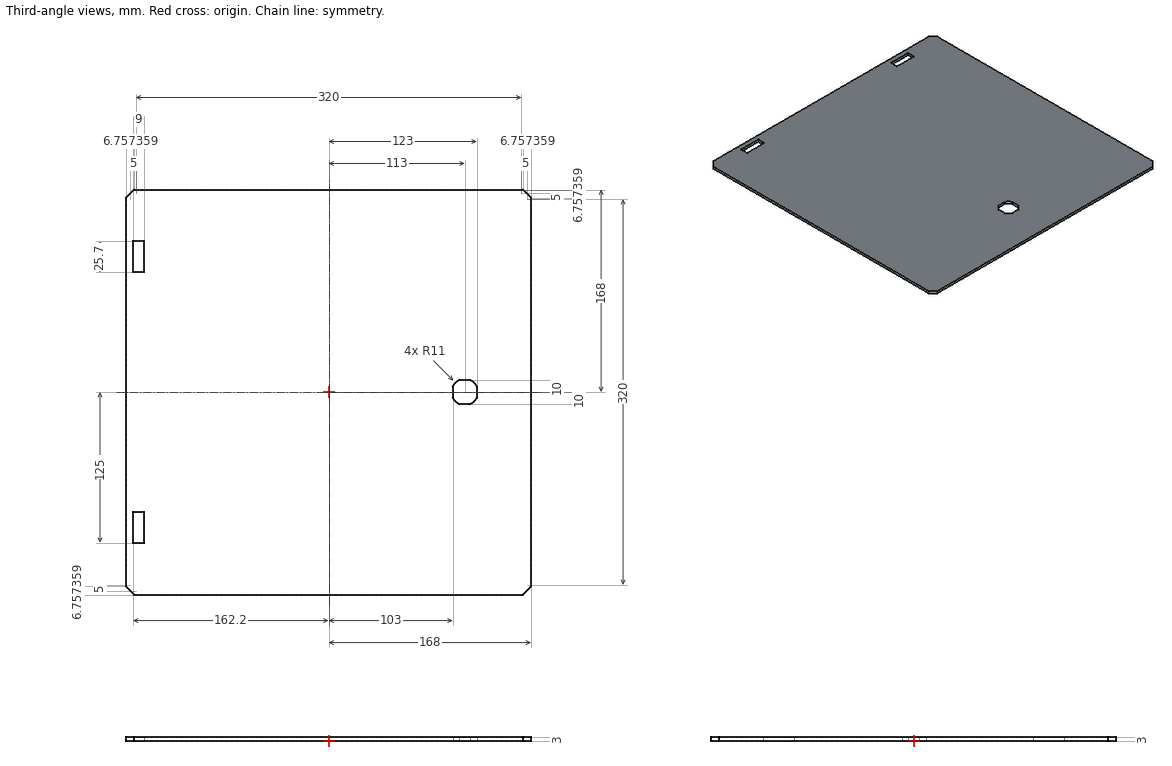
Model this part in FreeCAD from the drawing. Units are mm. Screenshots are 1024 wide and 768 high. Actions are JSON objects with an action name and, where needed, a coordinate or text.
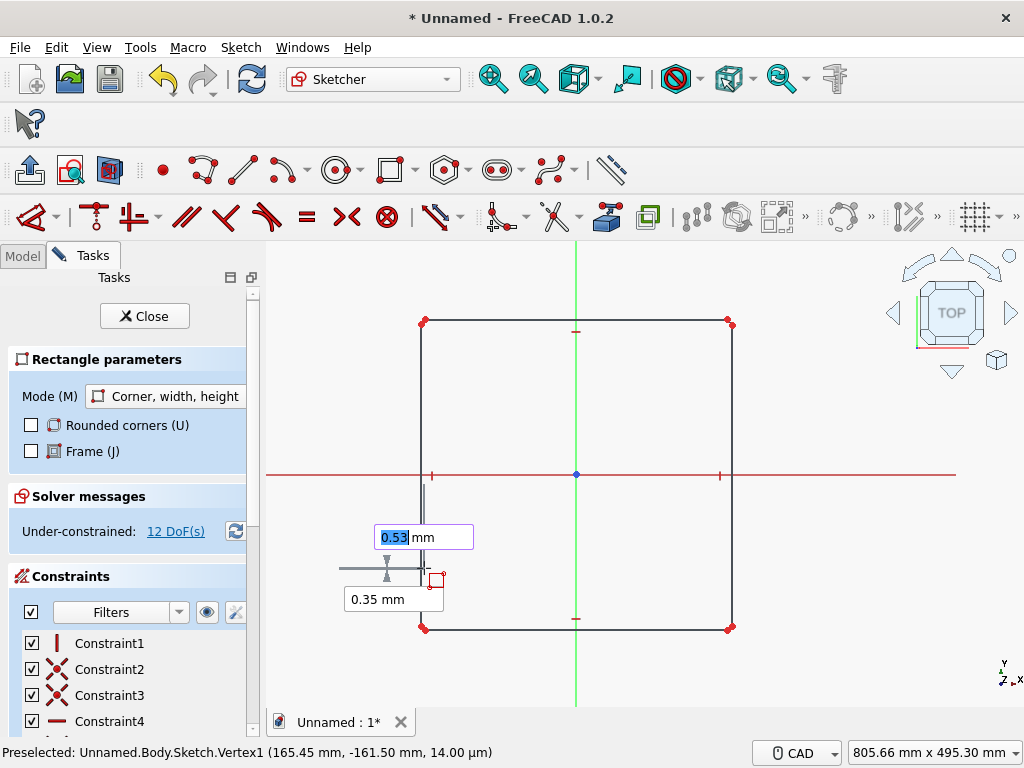
{"action": "scroll", "coordinate": [432, 592], "scroll_direction": "up", "scroll_amount": 2}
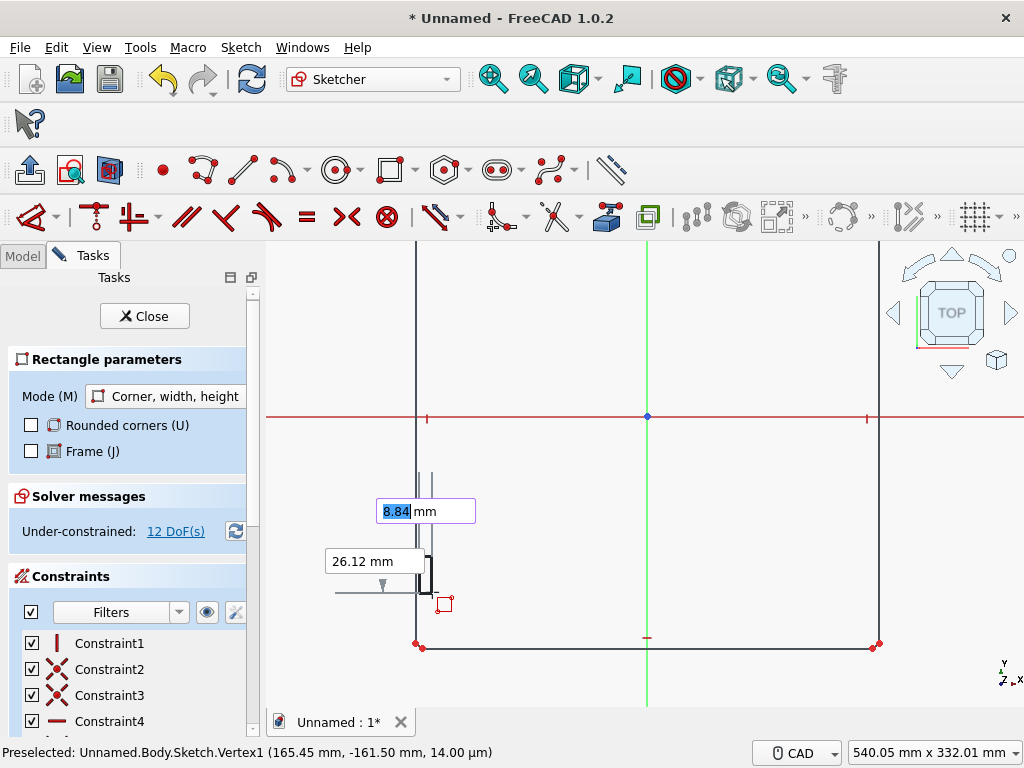
{"action": "left_click", "coordinate": [432, 592]}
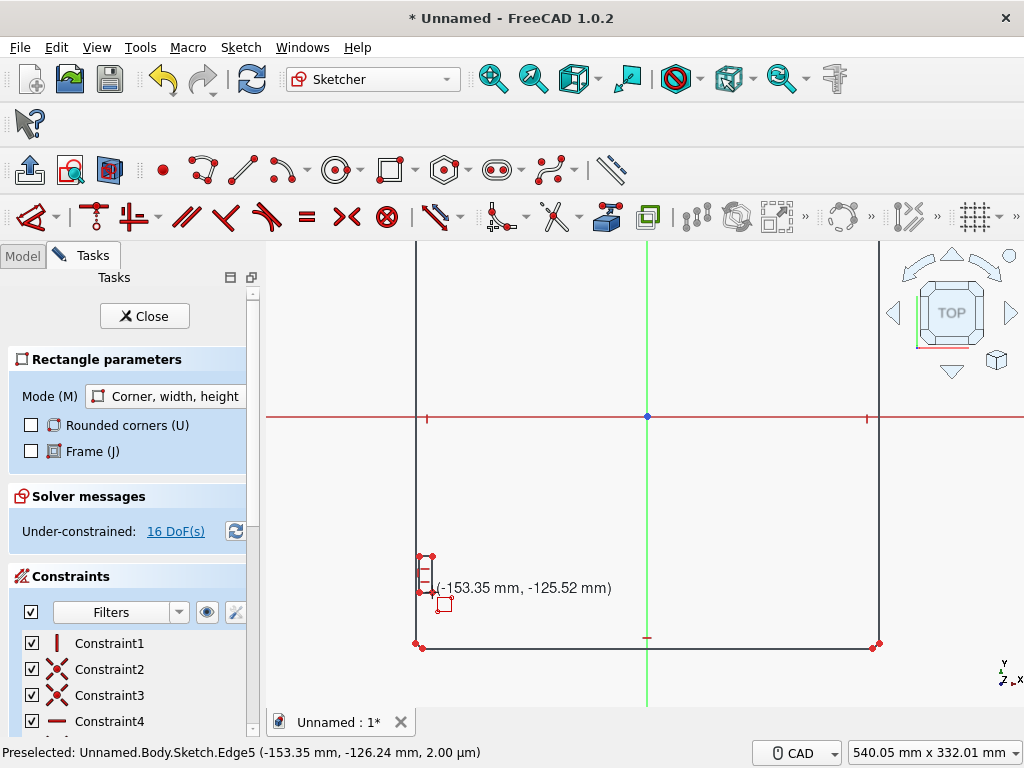
{"action": "scroll", "coordinate": [433, 590], "scroll_direction": "down", "scroll_amount": 2}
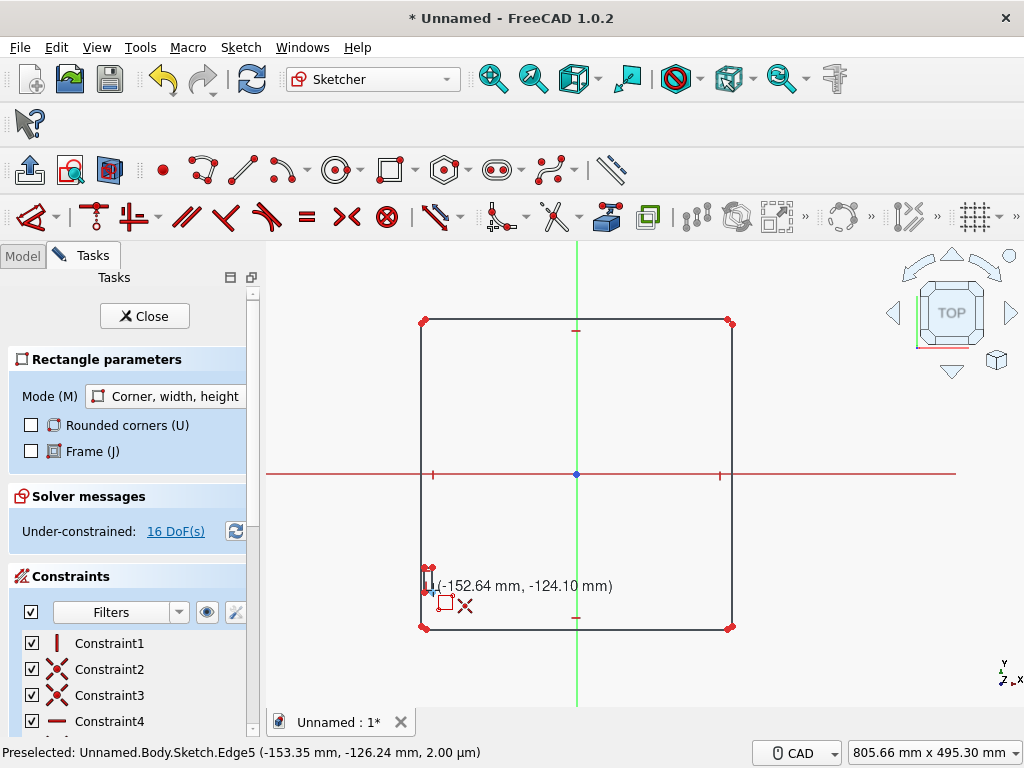
{"action": "scroll", "coordinate": [424, 357], "scroll_direction": "up", "scroll_amount": 9}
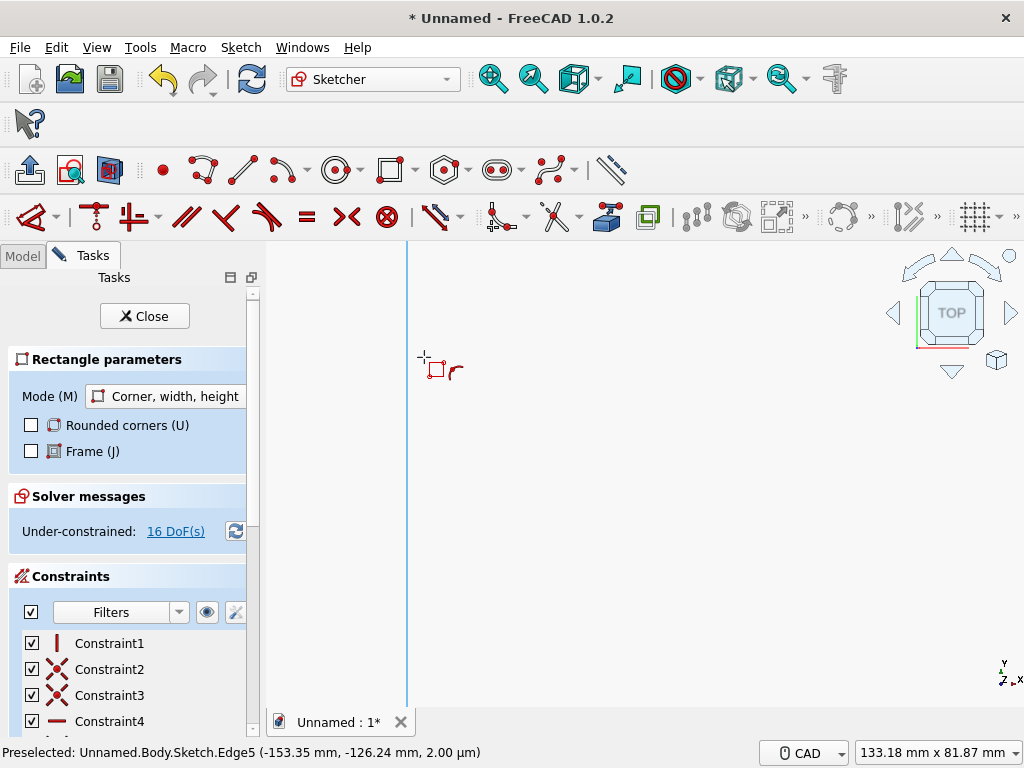
{"action": "left_click", "coordinate": [423, 353]}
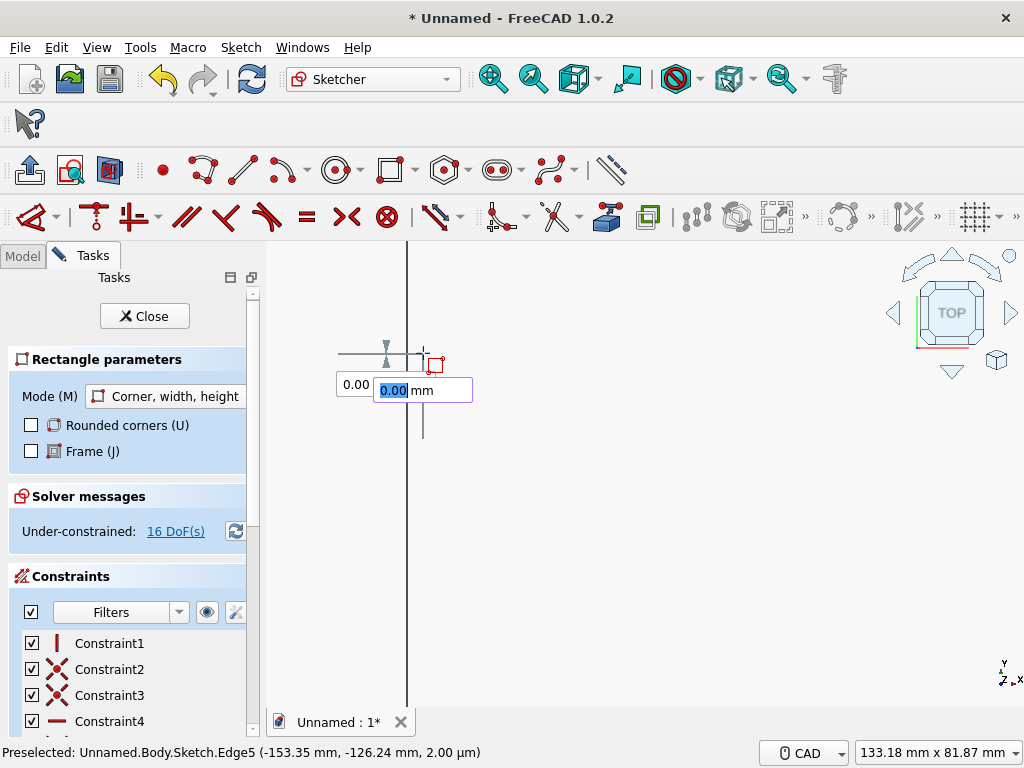
{"action": "scroll", "coordinate": [424, 357], "scroll_direction": "down", "scroll_amount": 9}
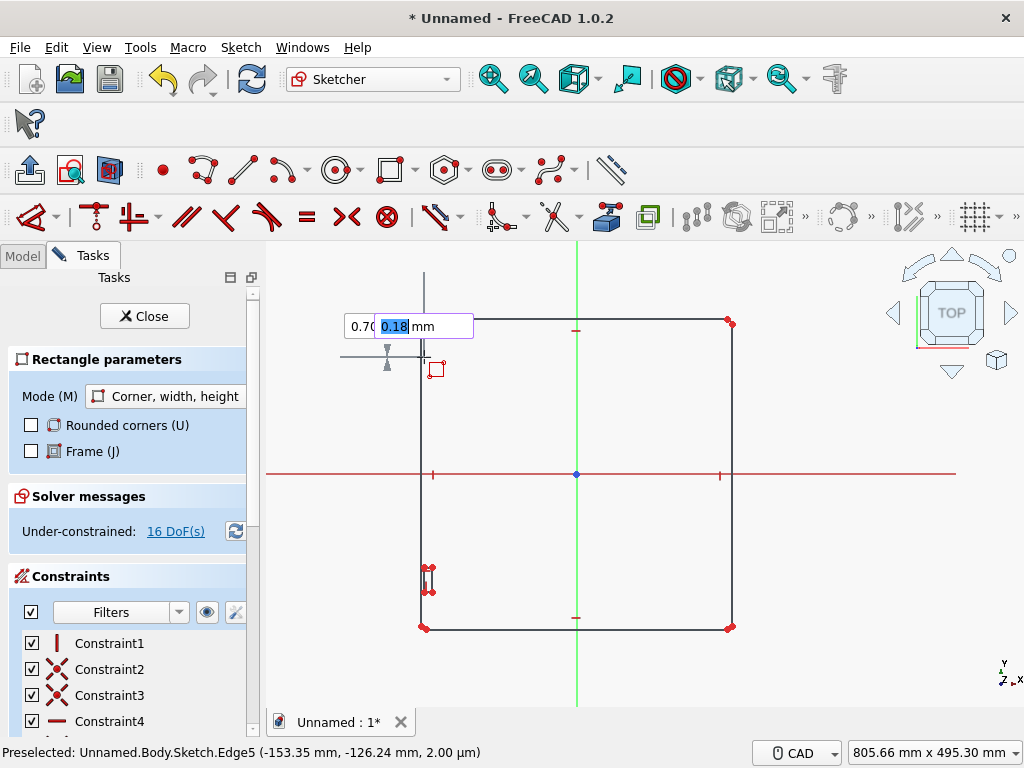
{"action": "scroll", "coordinate": [433, 381], "scroll_direction": "up", "scroll_amount": 2}
{"action": "mouse_move", "coordinate": [432, 380]}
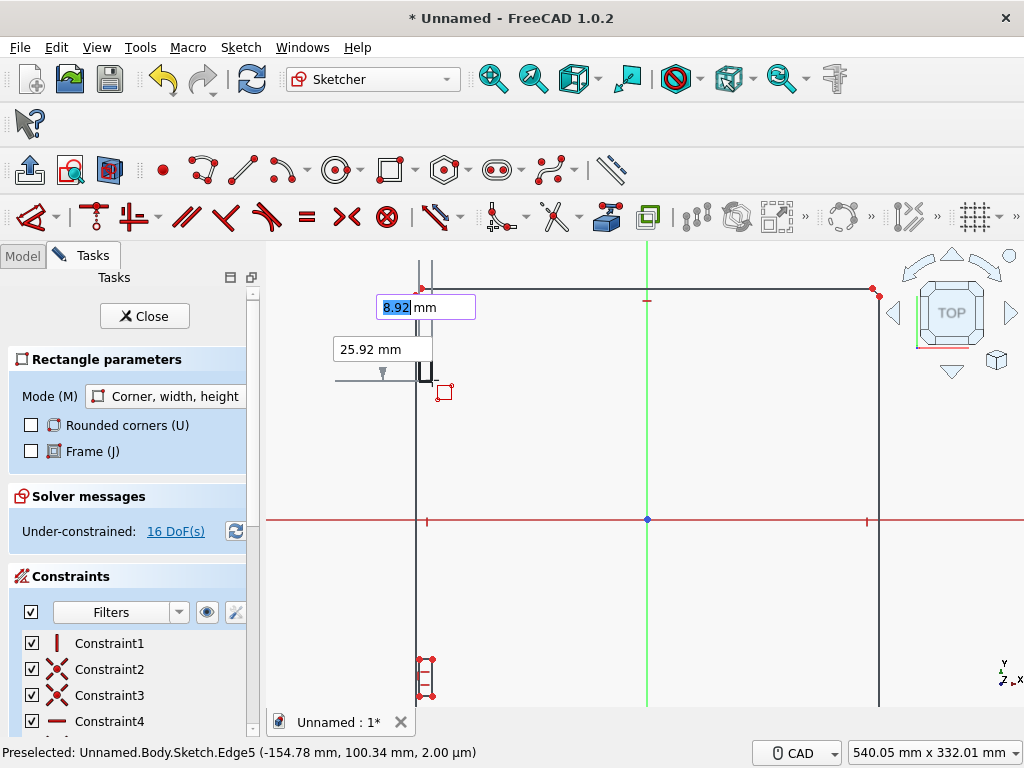
{"action": "type", "text": "9"}
{"action": "key", "text": "Tab"}
{"action": "type", "text": "25.7"}
{"action": "key", "text": "Return"}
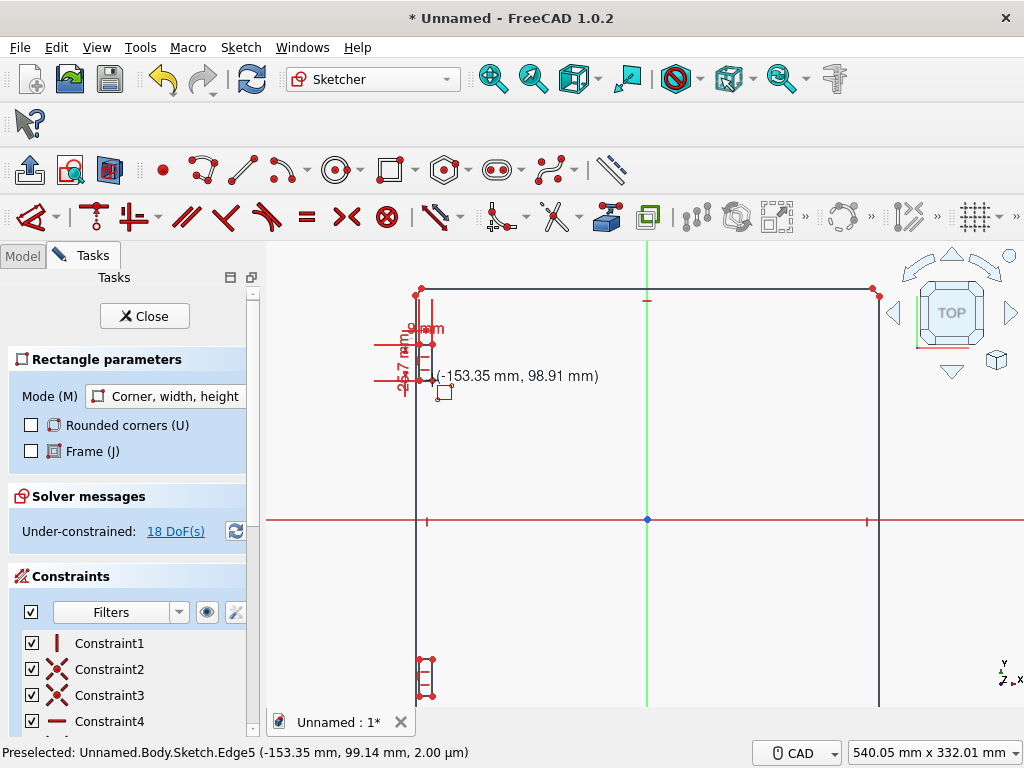
{"action": "left_click", "coordinate": [244, 170]}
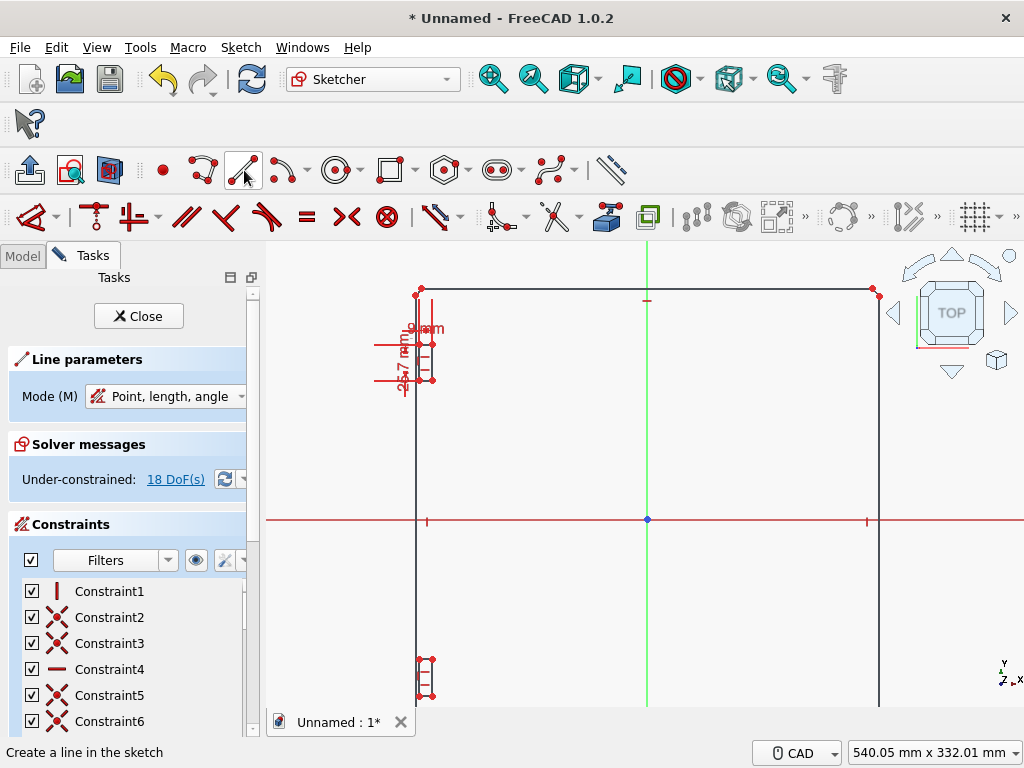
{"action": "left_click", "coordinate": [799, 506]}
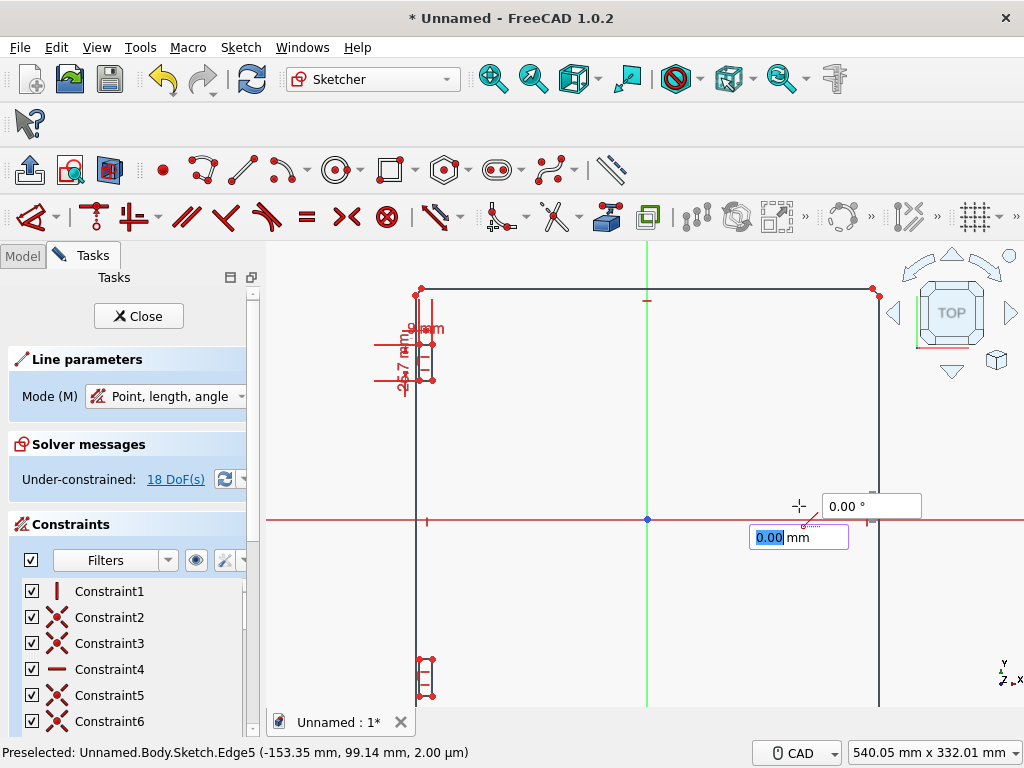
{"action": "scroll", "coordinate": [812, 506], "scroll_direction": "up", "scroll_amount": 2}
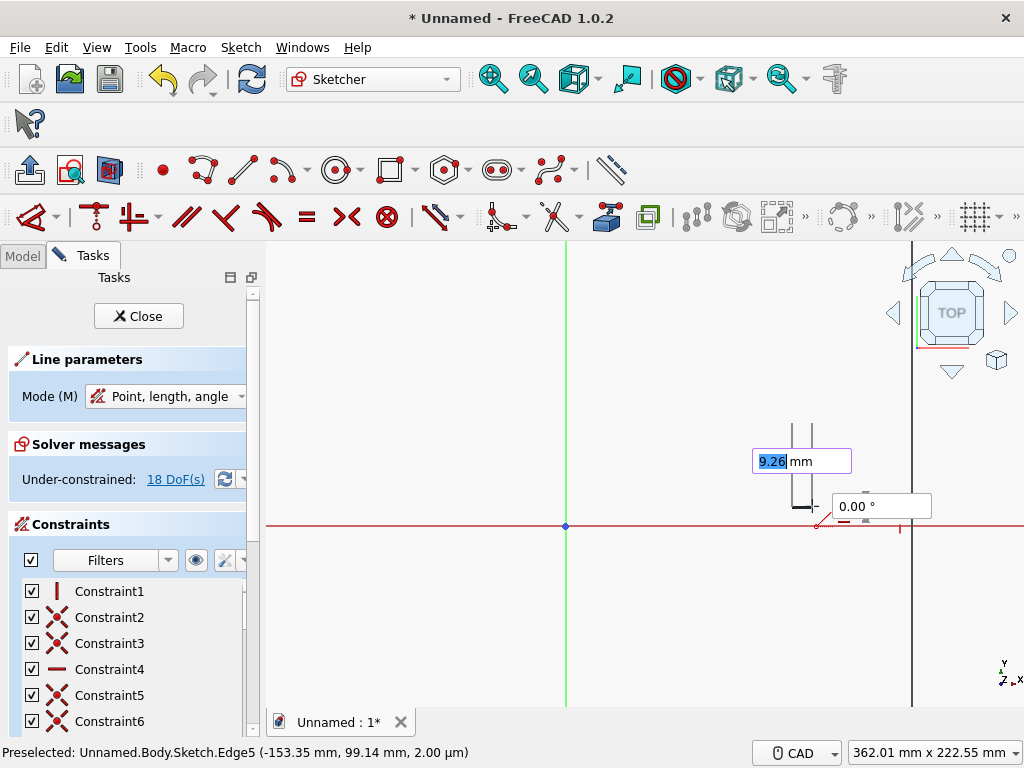
{"action": "left_click", "coordinate": [812, 506]}